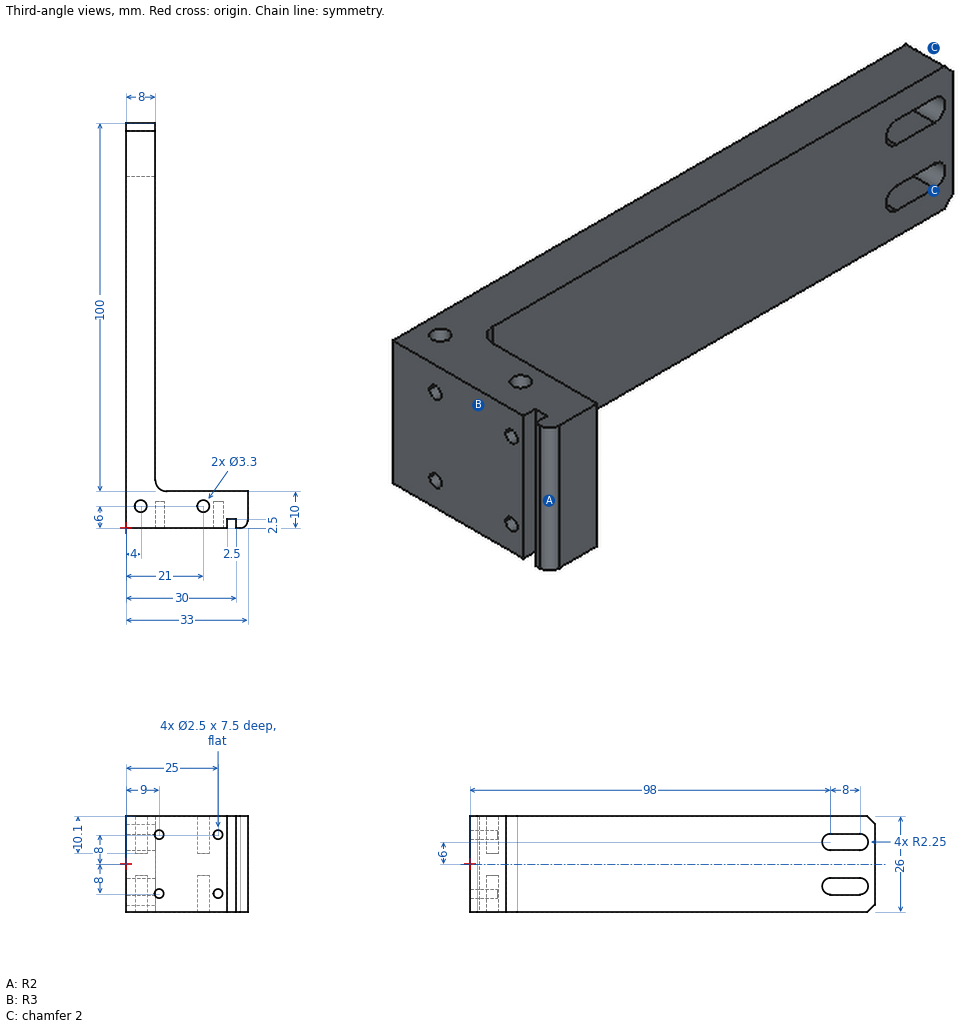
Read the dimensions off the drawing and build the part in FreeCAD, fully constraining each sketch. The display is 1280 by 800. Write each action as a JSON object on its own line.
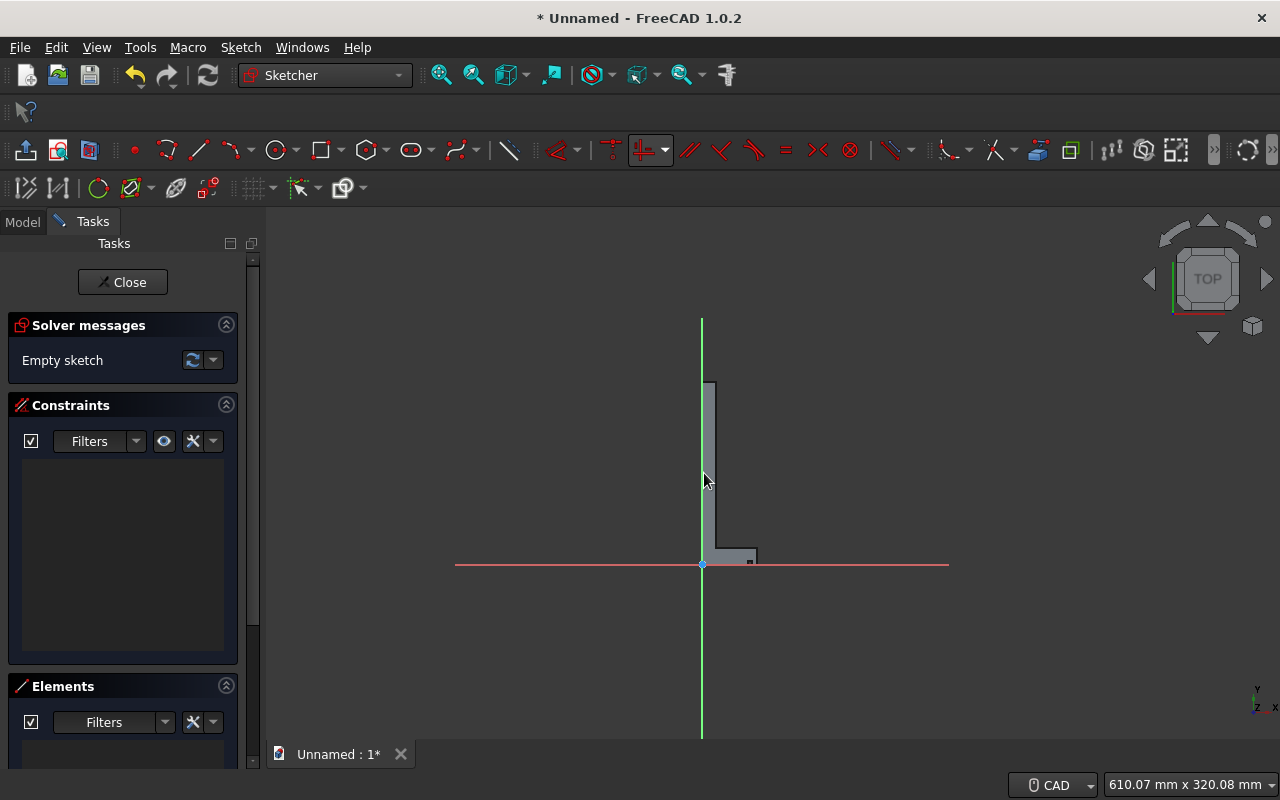
{"action": "scroll", "coordinate": [722, 564], "scroll_direction": "up", "scroll_amount": 14}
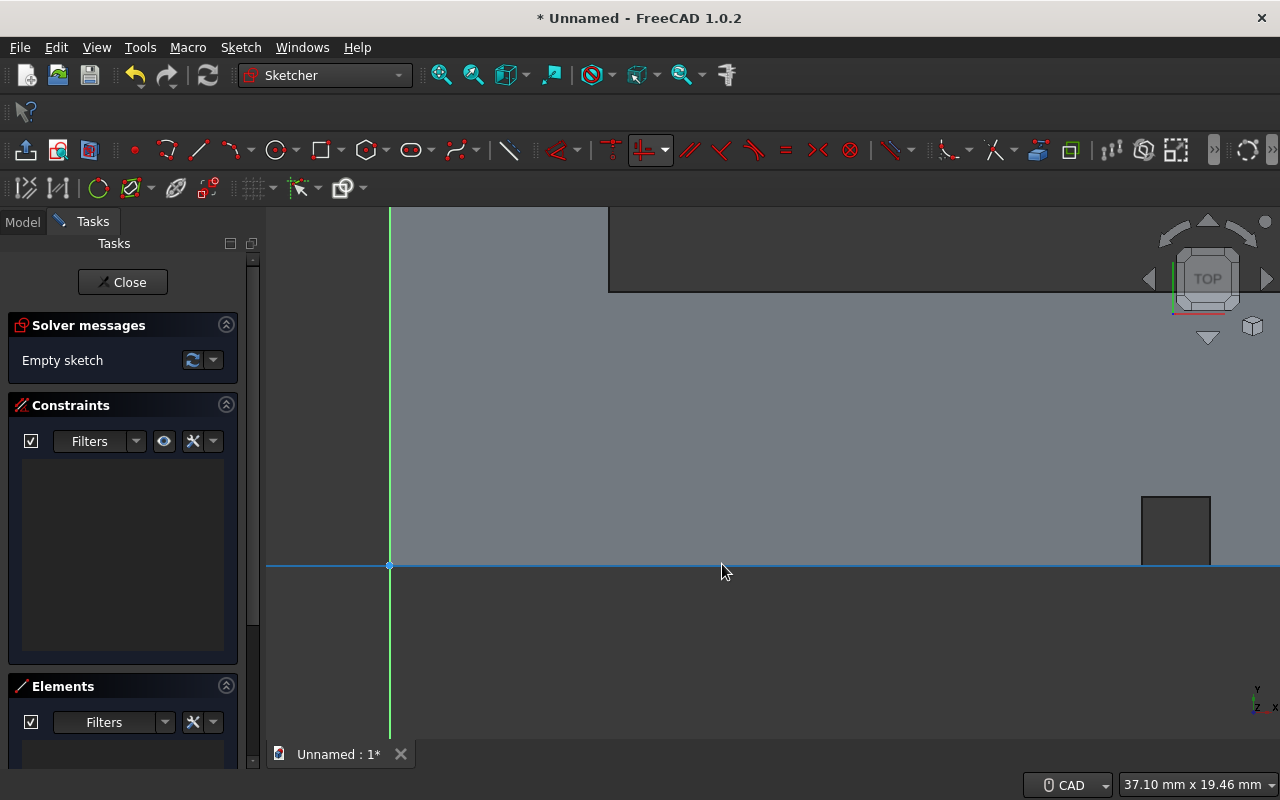
{"action": "left_click", "coordinate": [276, 150]}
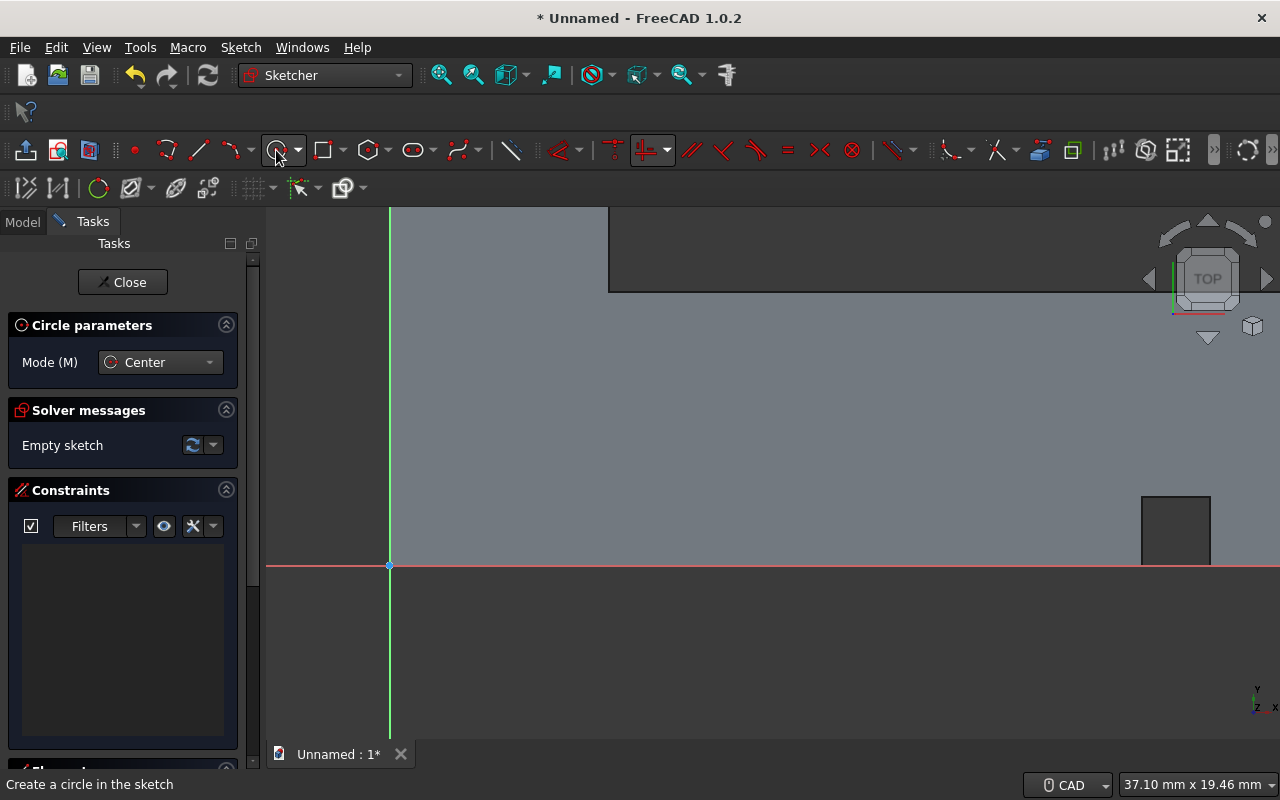
{"action": "left_click", "coordinate": [964, 402]}
{"action": "mouse_move", "coordinate": [996, 370]}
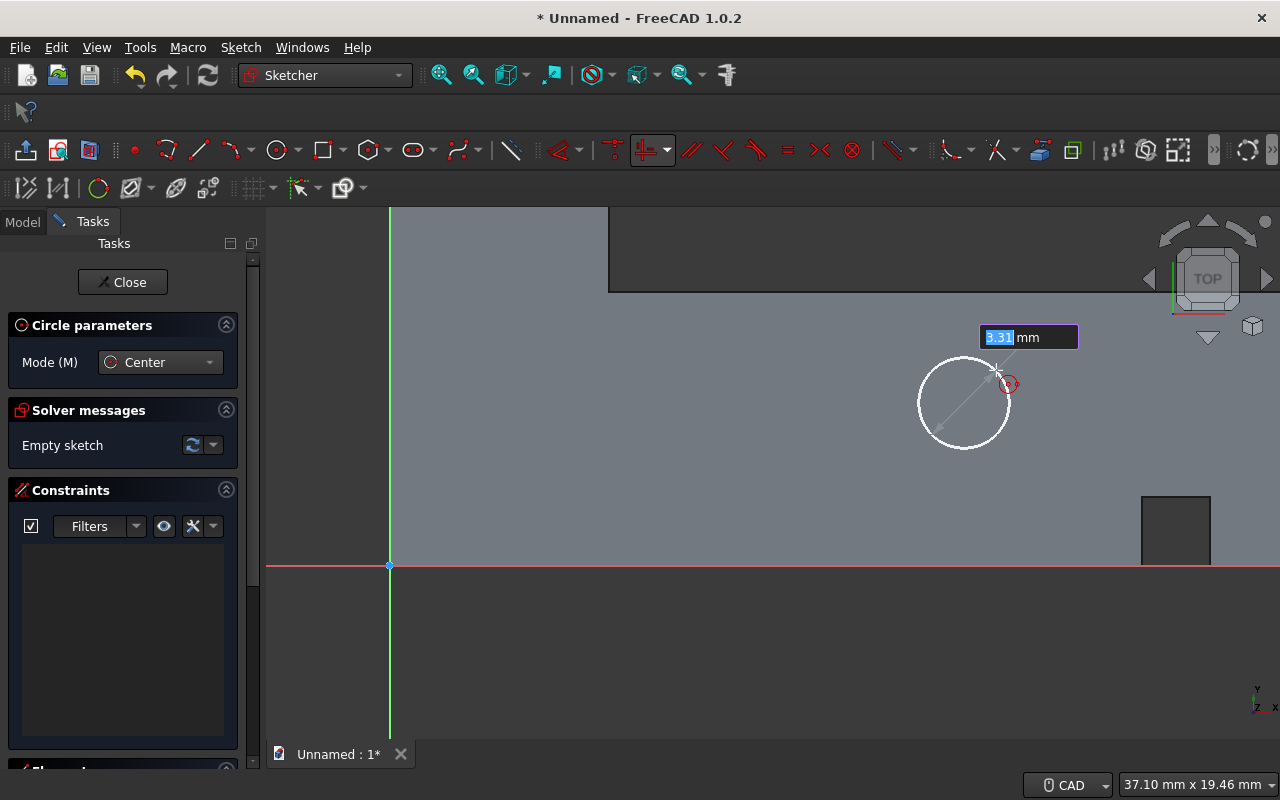
{"action": "type", "text": "3.3"}
{"action": "key", "text": "Return"}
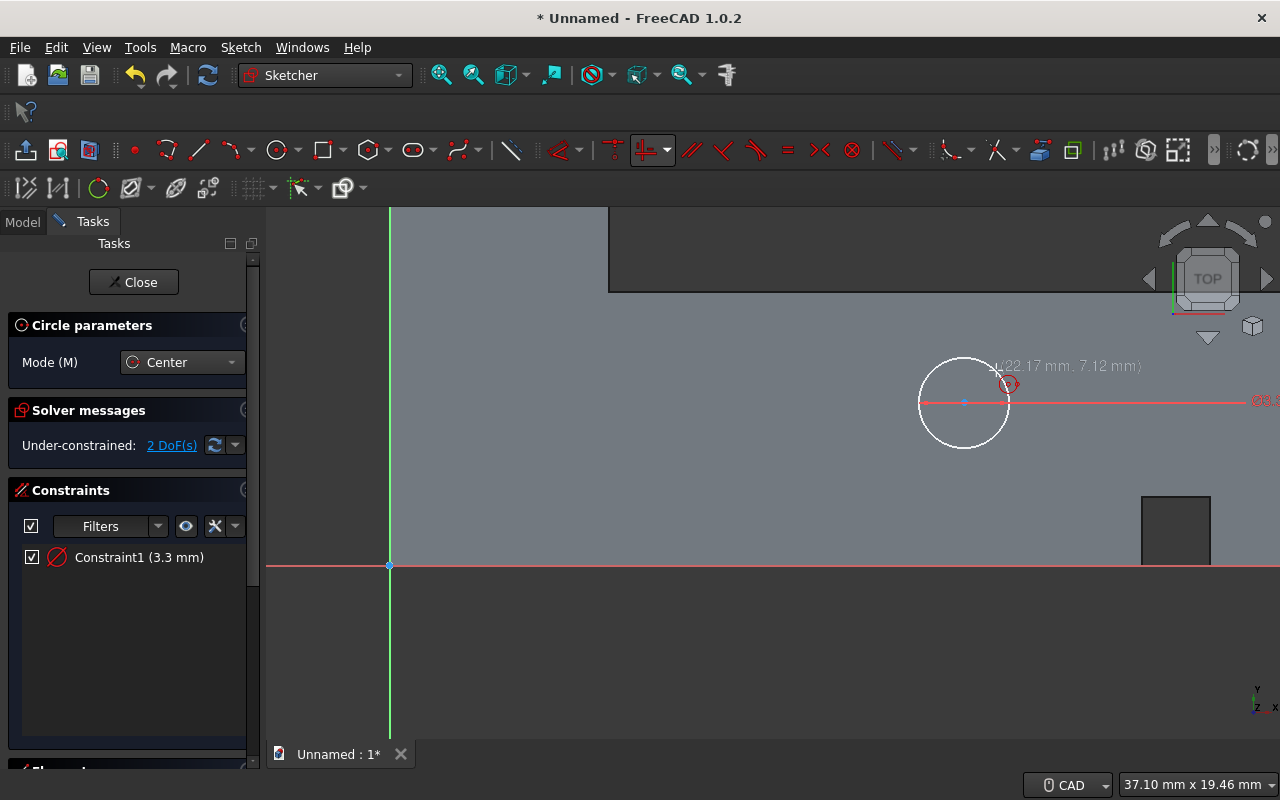
{"action": "left_click", "coordinate": [499, 402]}
{"action": "mouse_move", "coordinate": [531, 370]}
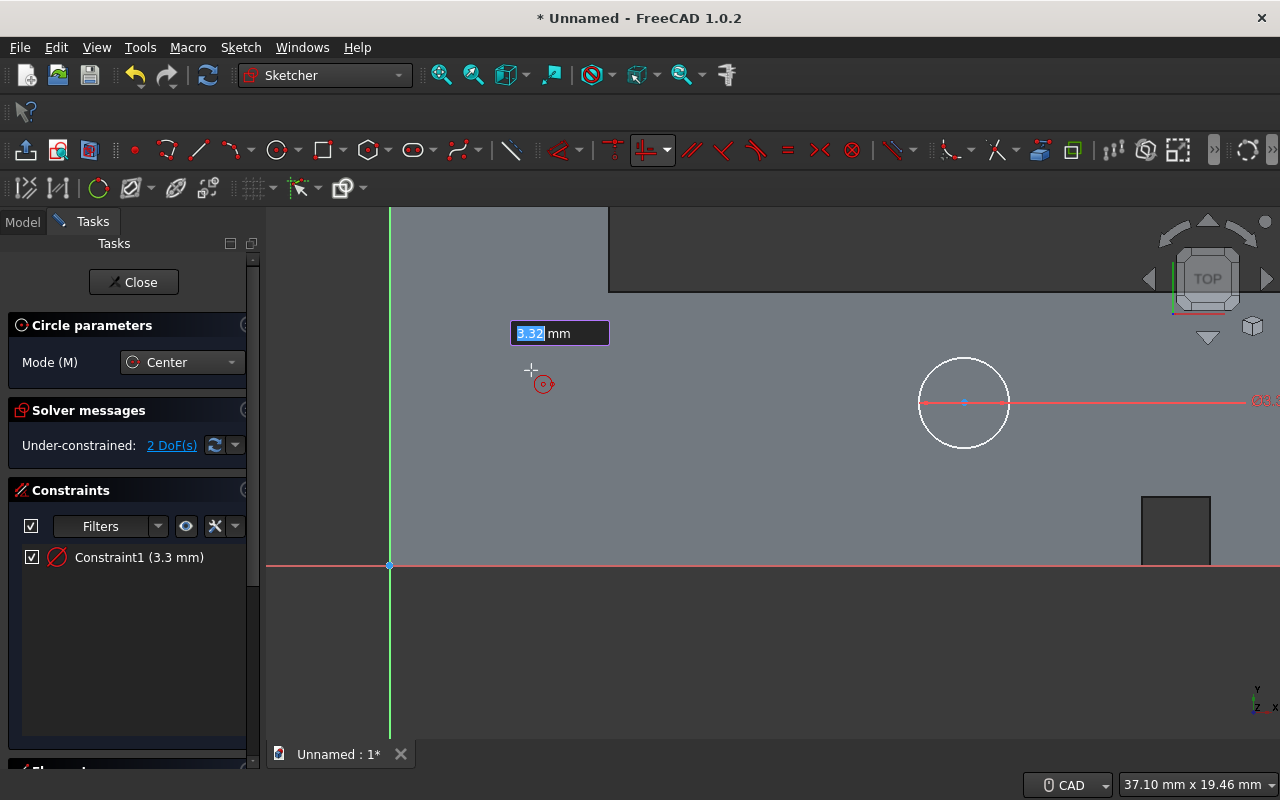
{"action": "type", "text": "3.3"}
{"action": "key", "text": "Return"}
{"action": "key", "text": "Escape"}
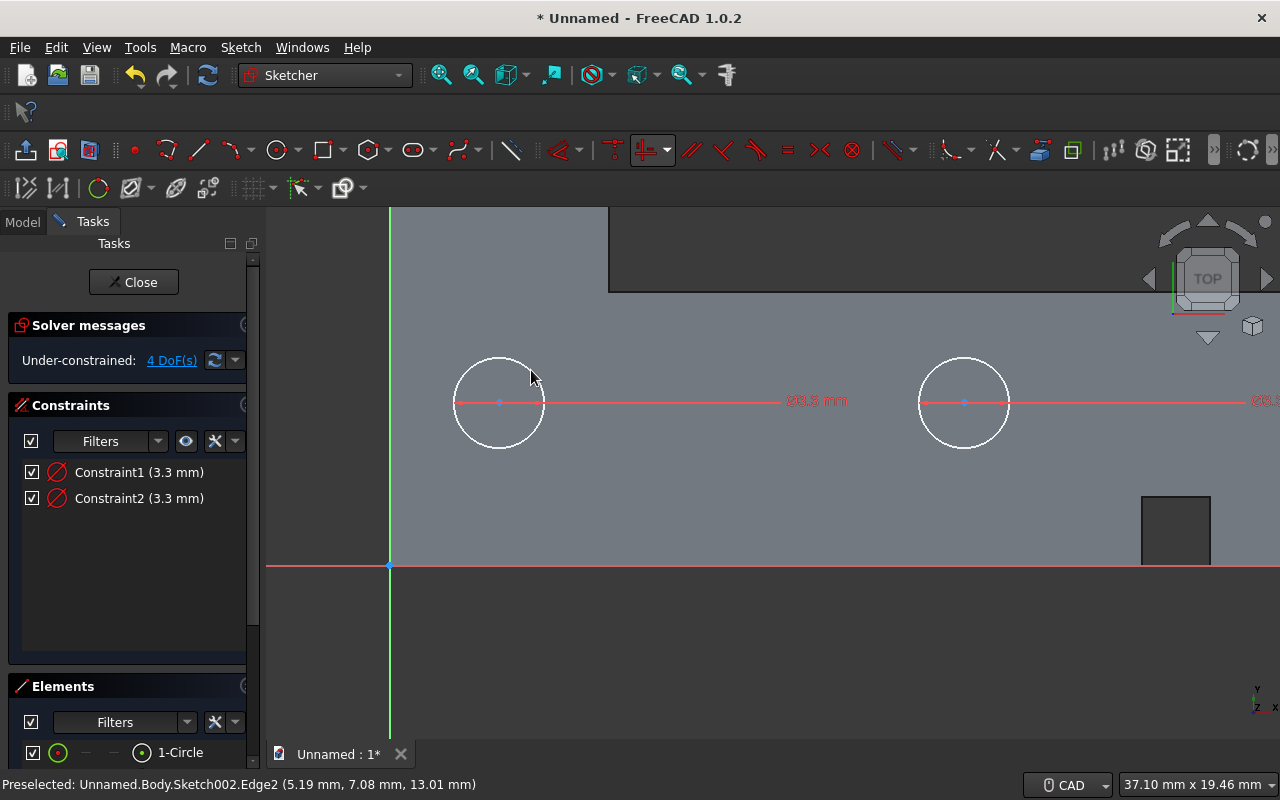
{"action": "left_click", "coordinate": [964, 403]}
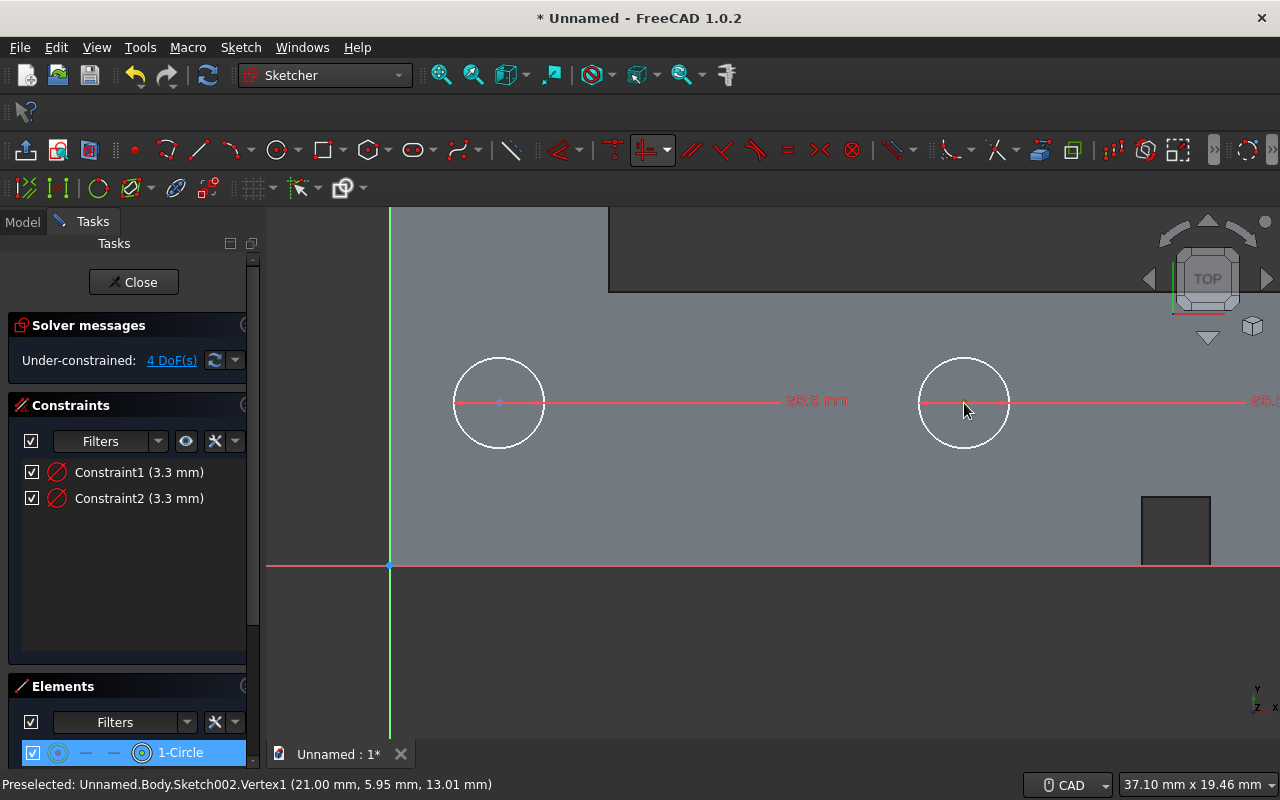
{"action": "left_click", "coordinate": [499, 403]}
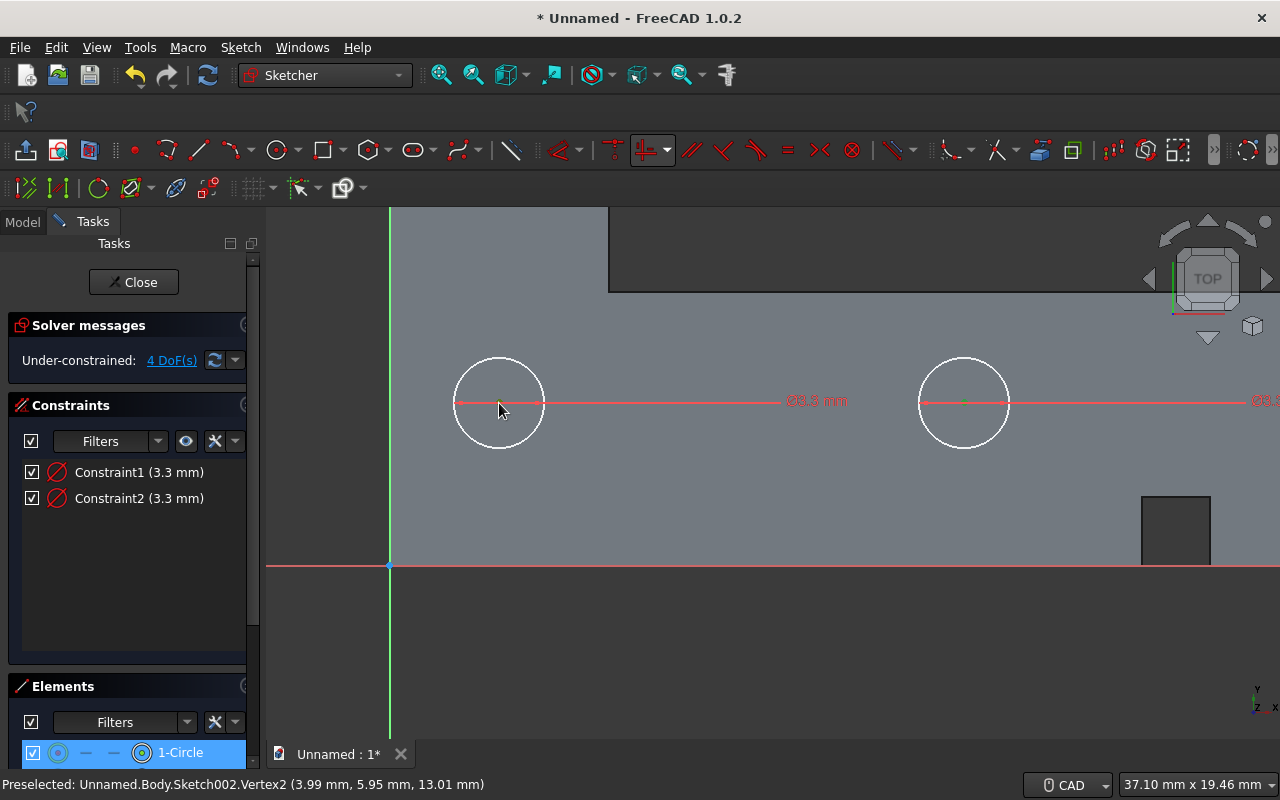
{"action": "key", "text": "h"}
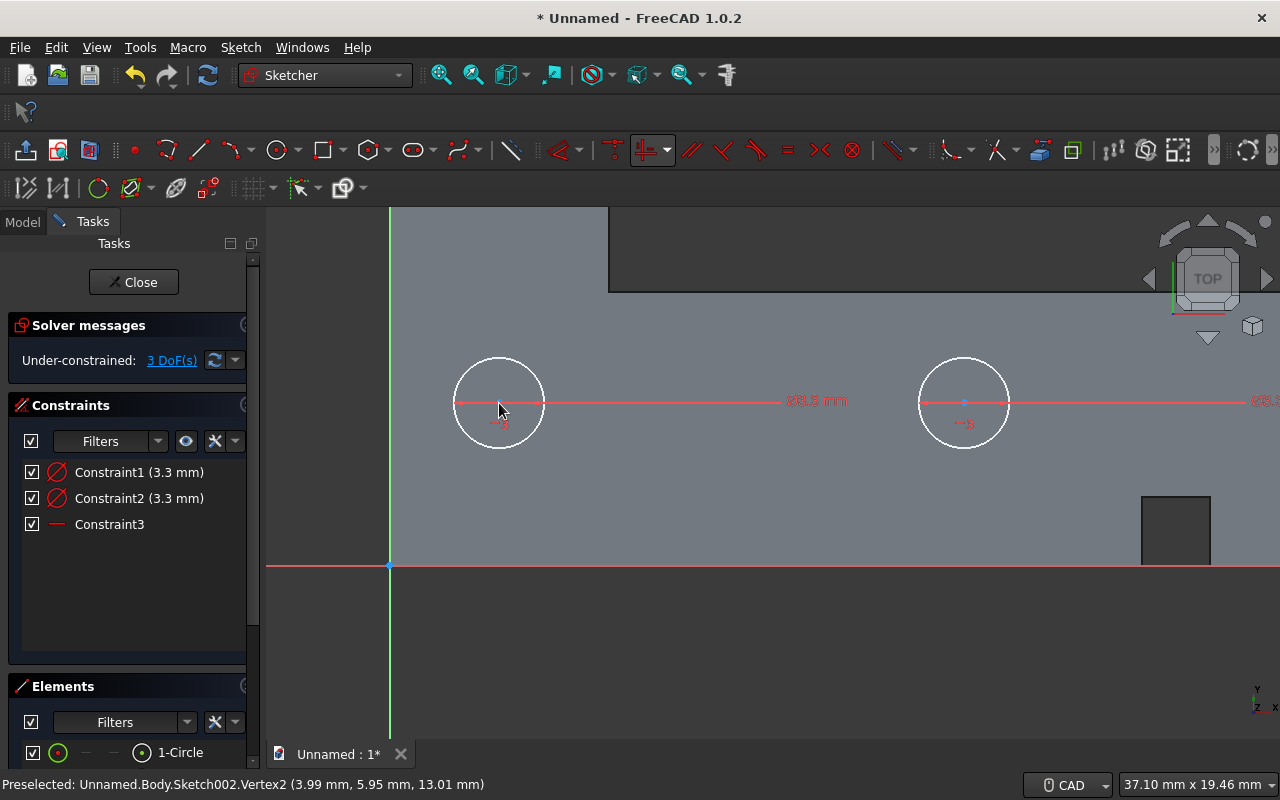
{"action": "left_click", "coordinate": [558, 150]}